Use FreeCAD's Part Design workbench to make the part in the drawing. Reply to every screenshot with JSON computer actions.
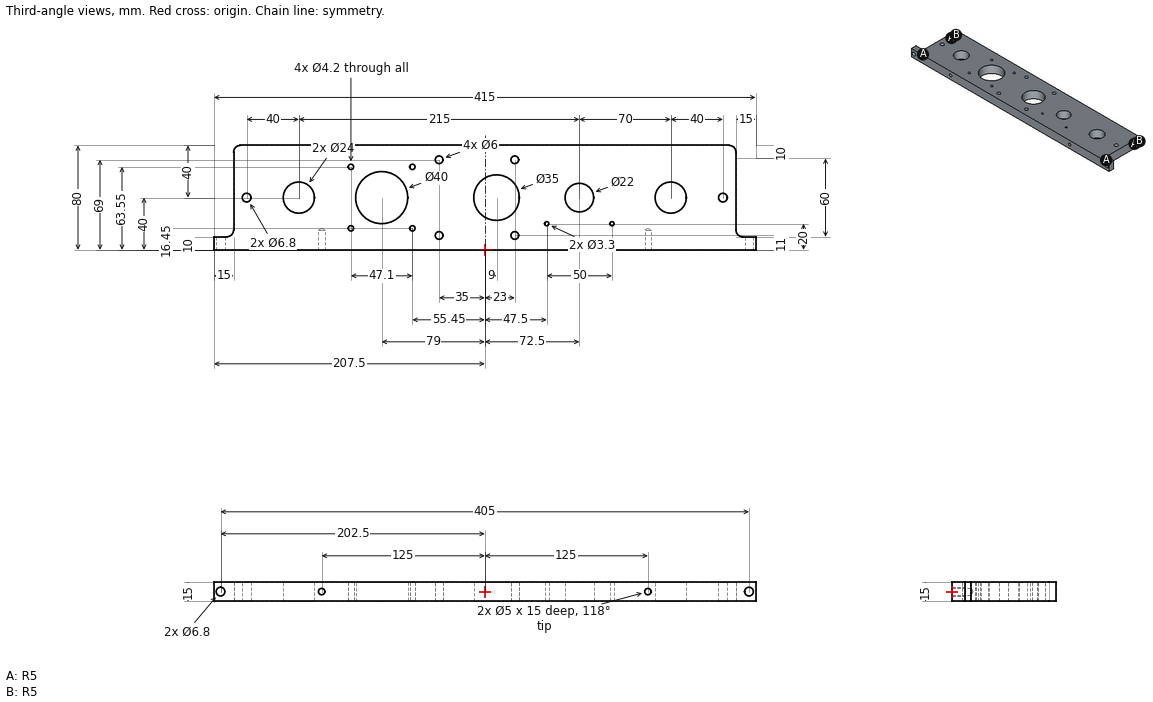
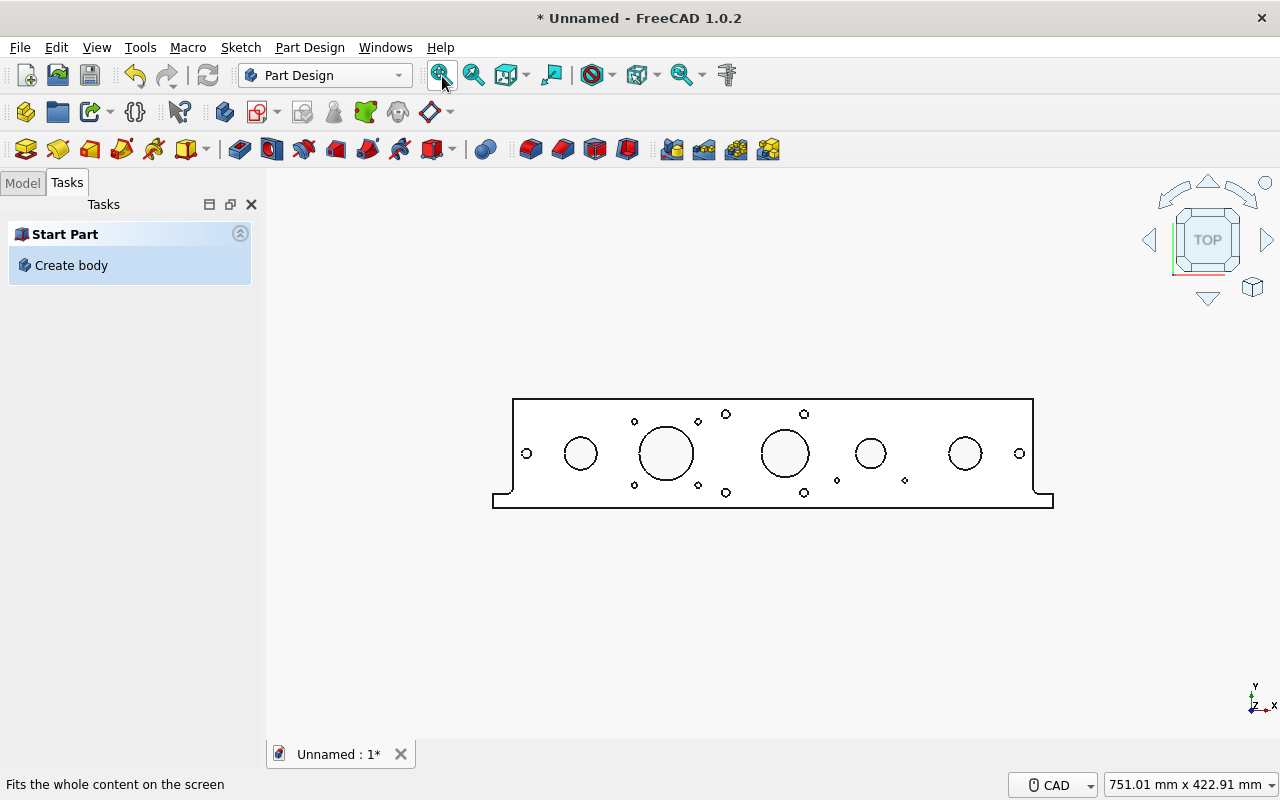
{"action": "key", "text": "0"}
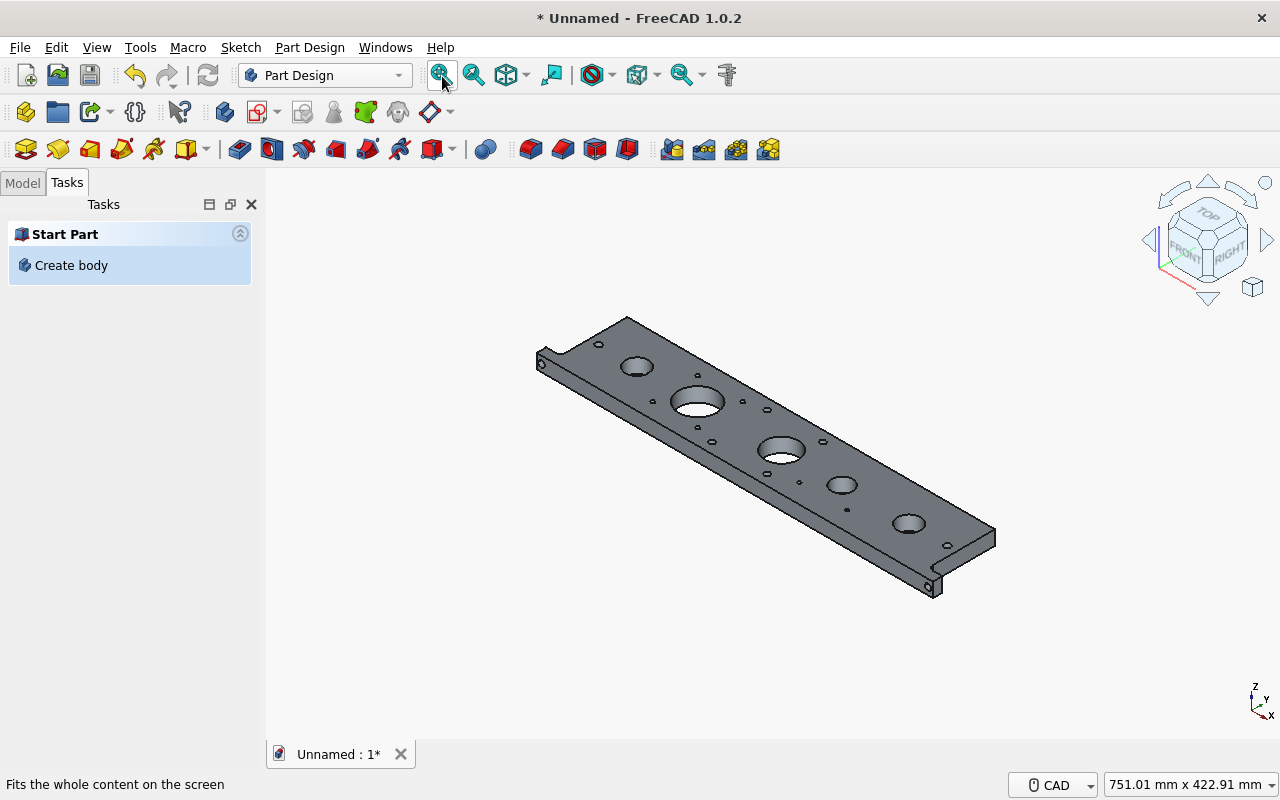
{"action": "scroll", "coordinate": [627, 324], "scroll_direction": "up", "scroll_amount": 4}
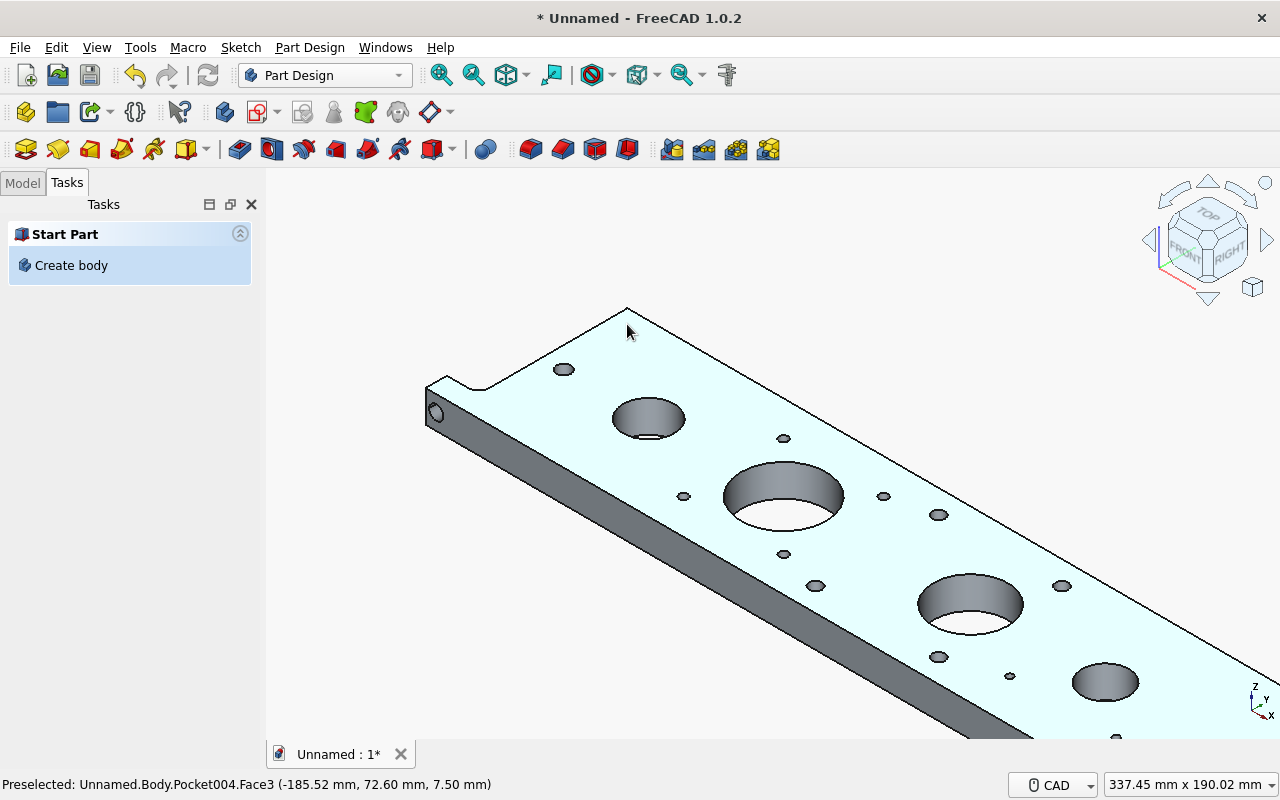
{"action": "left_click", "coordinate": [442, 76]}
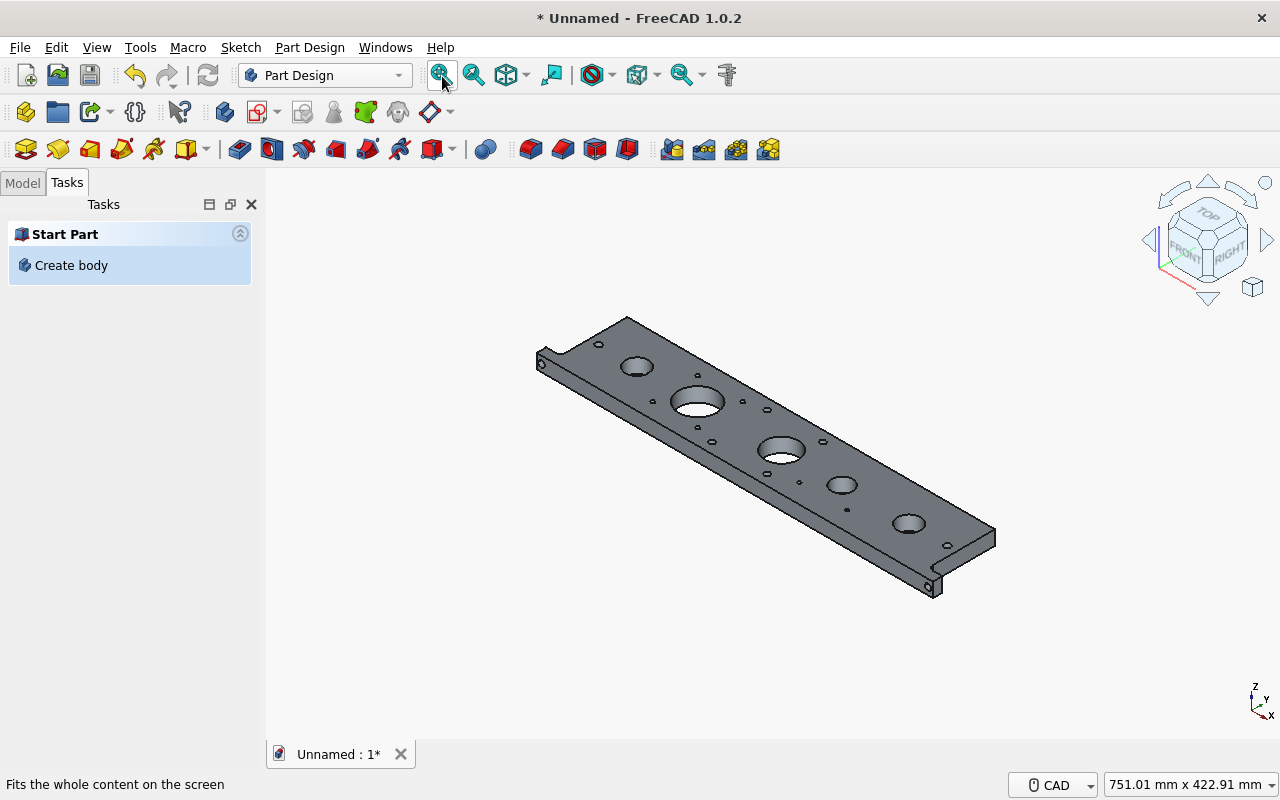
{"action": "key", "text": "1"}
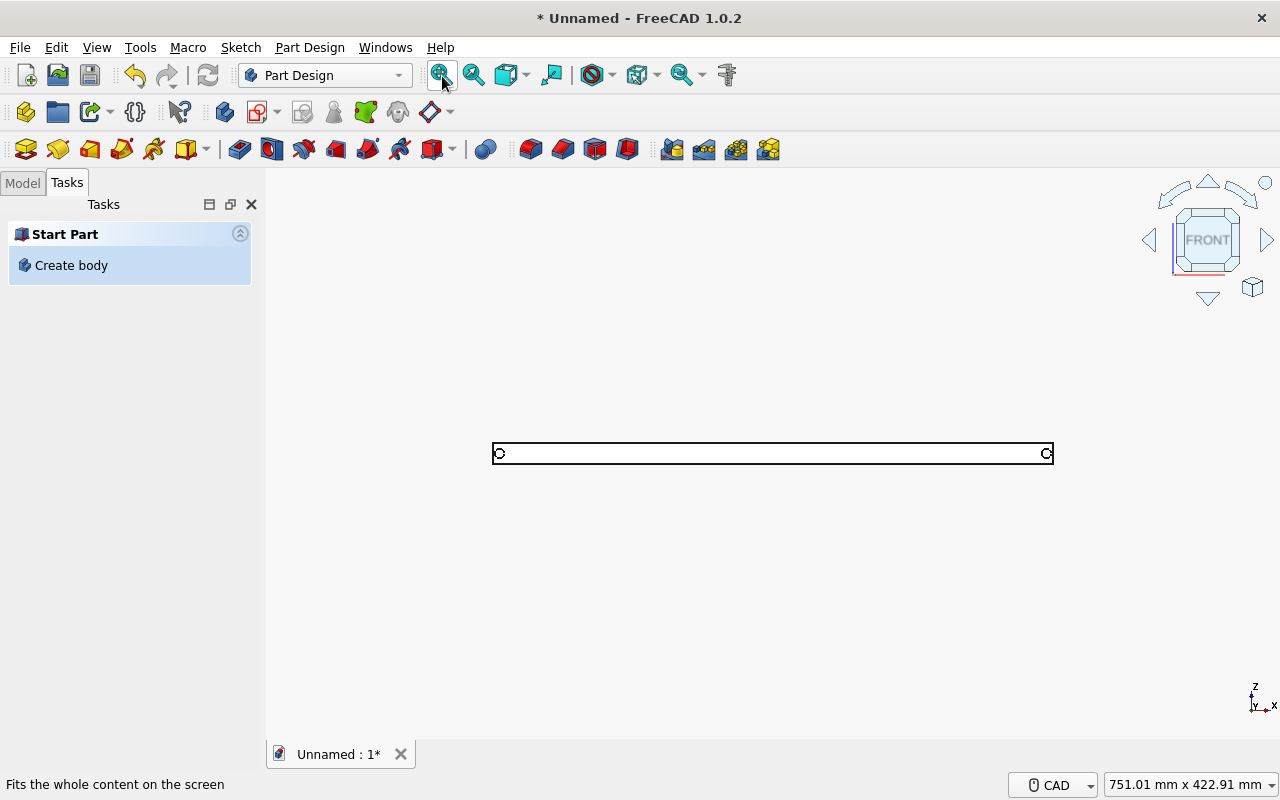
{"action": "scroll", "coordinate": [513, 452], "scroll_direction": "up", "scroll_amount": 4}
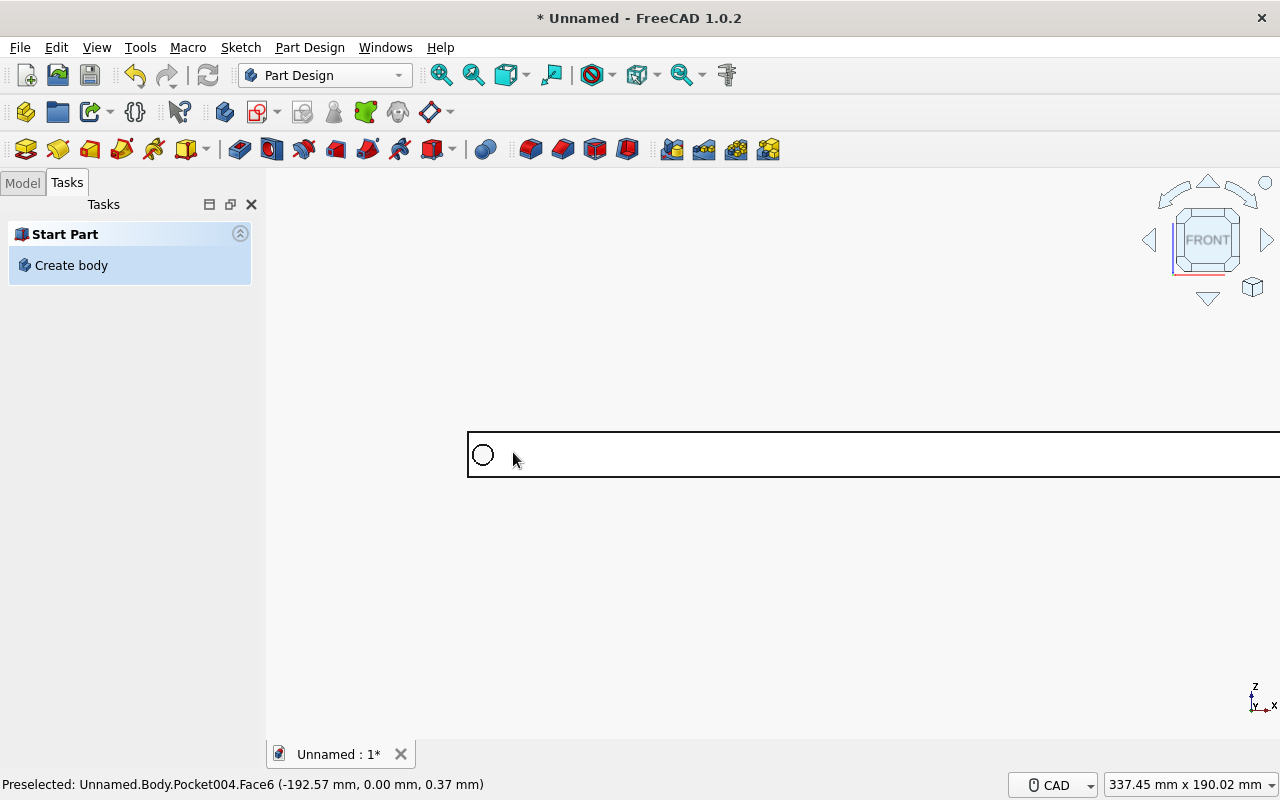
{"action": "left_click", "coordinate": [442, 76]}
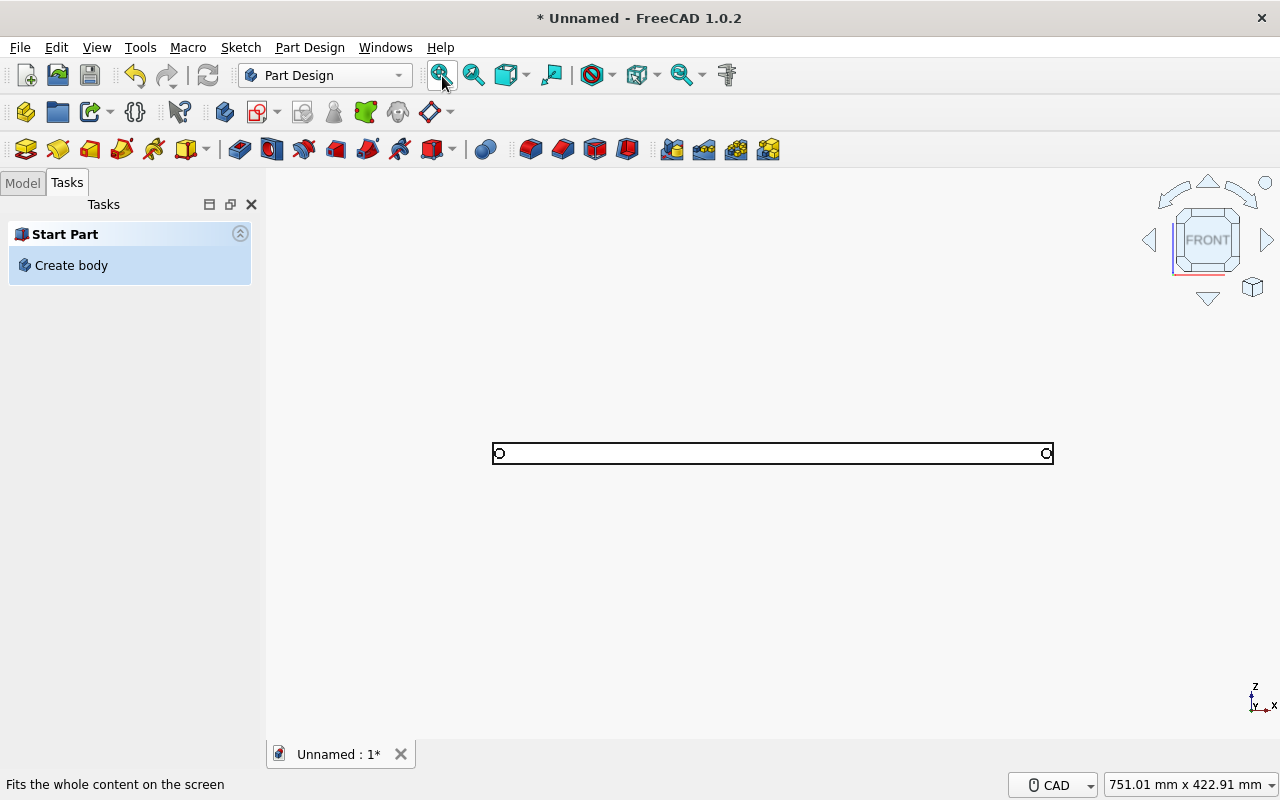
{"action": "key", "text": "3"}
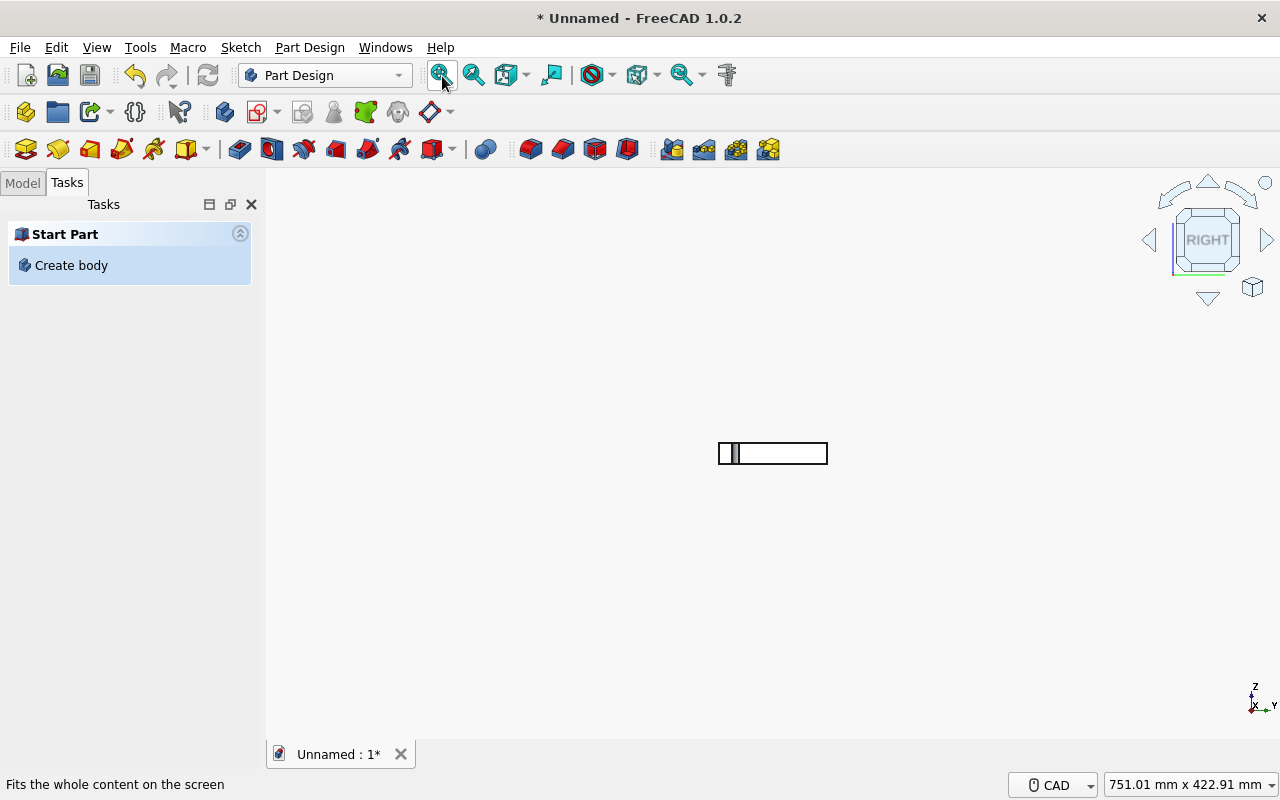
{"action": "left_click", "coordinate": [442, 76]}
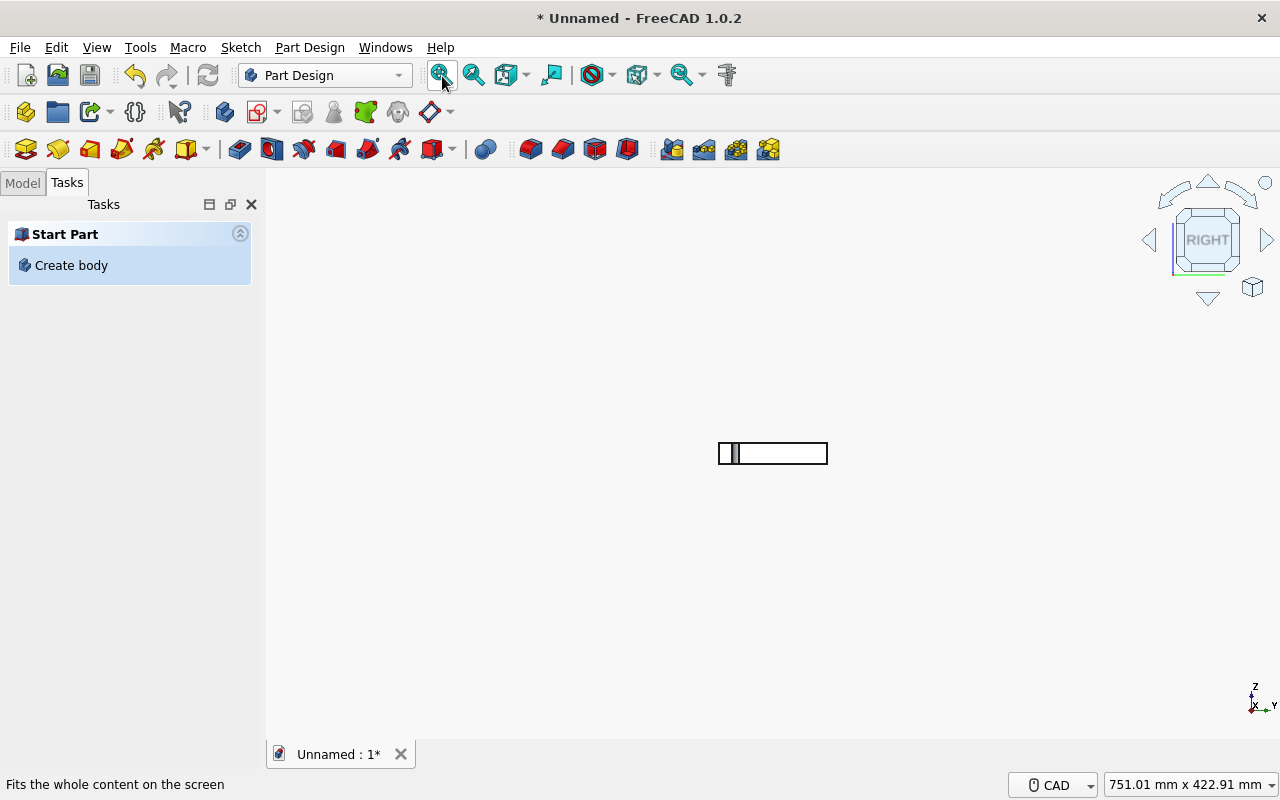
{"action": "left_click", "coordinate": [827, 452]}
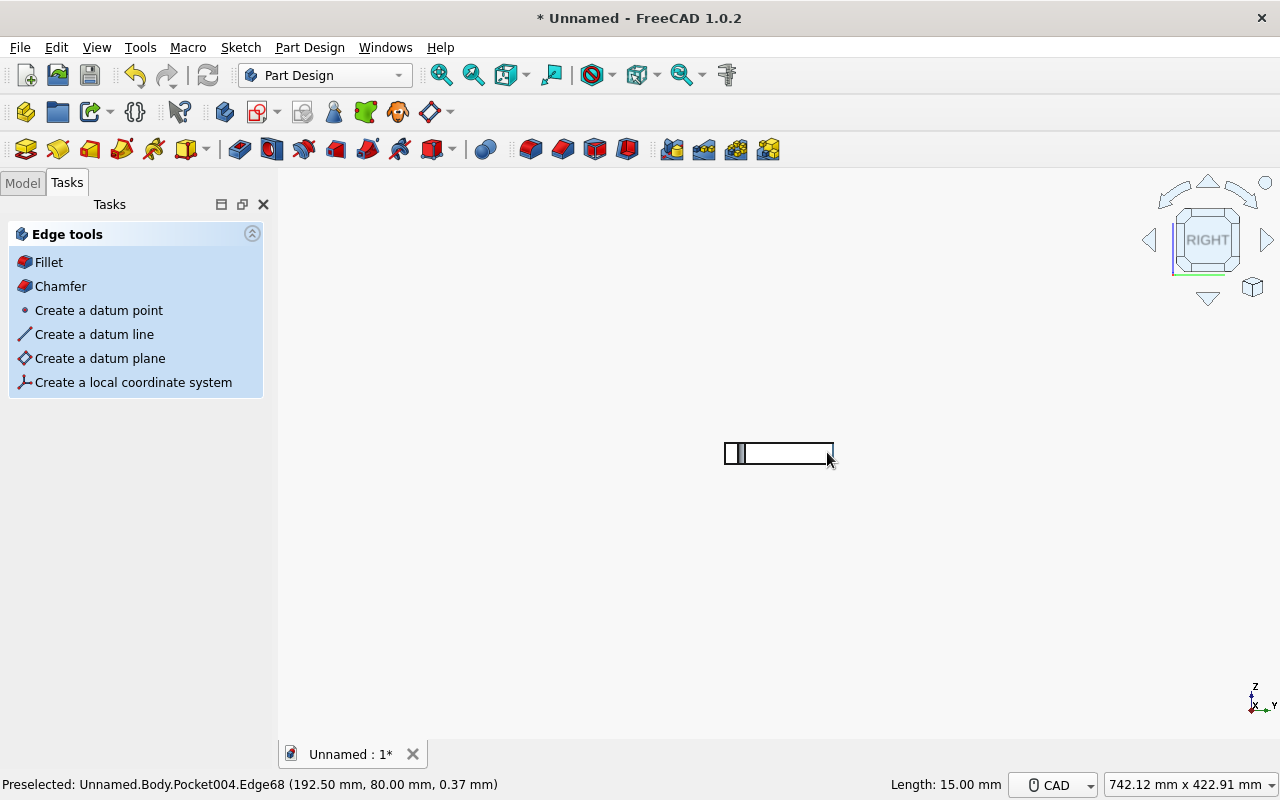
{"action": "scroll", "coordinate": [833, 452], "scroll_direction": "up", "scroll_amount": 4}